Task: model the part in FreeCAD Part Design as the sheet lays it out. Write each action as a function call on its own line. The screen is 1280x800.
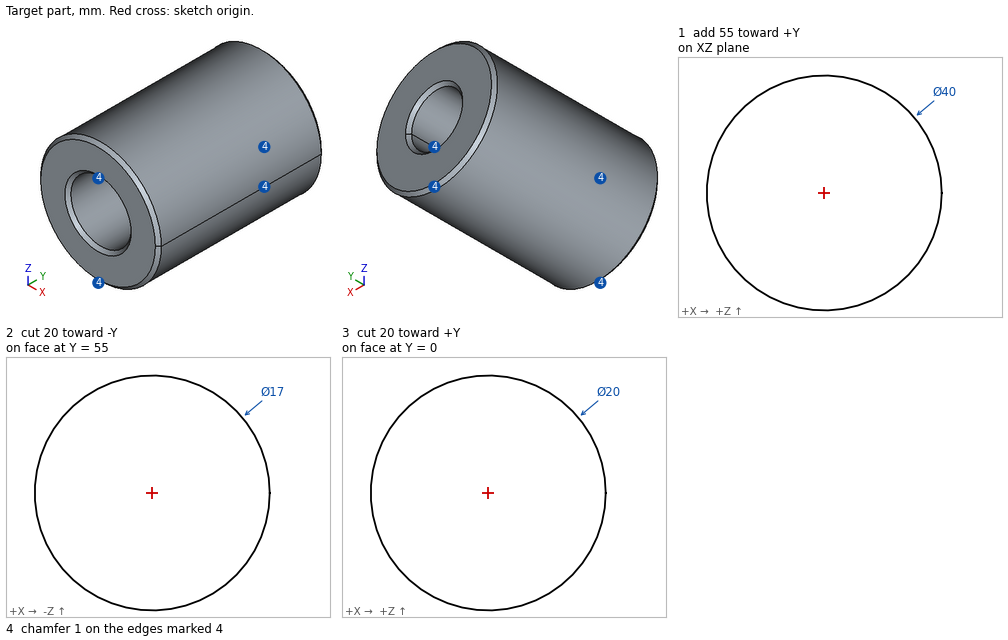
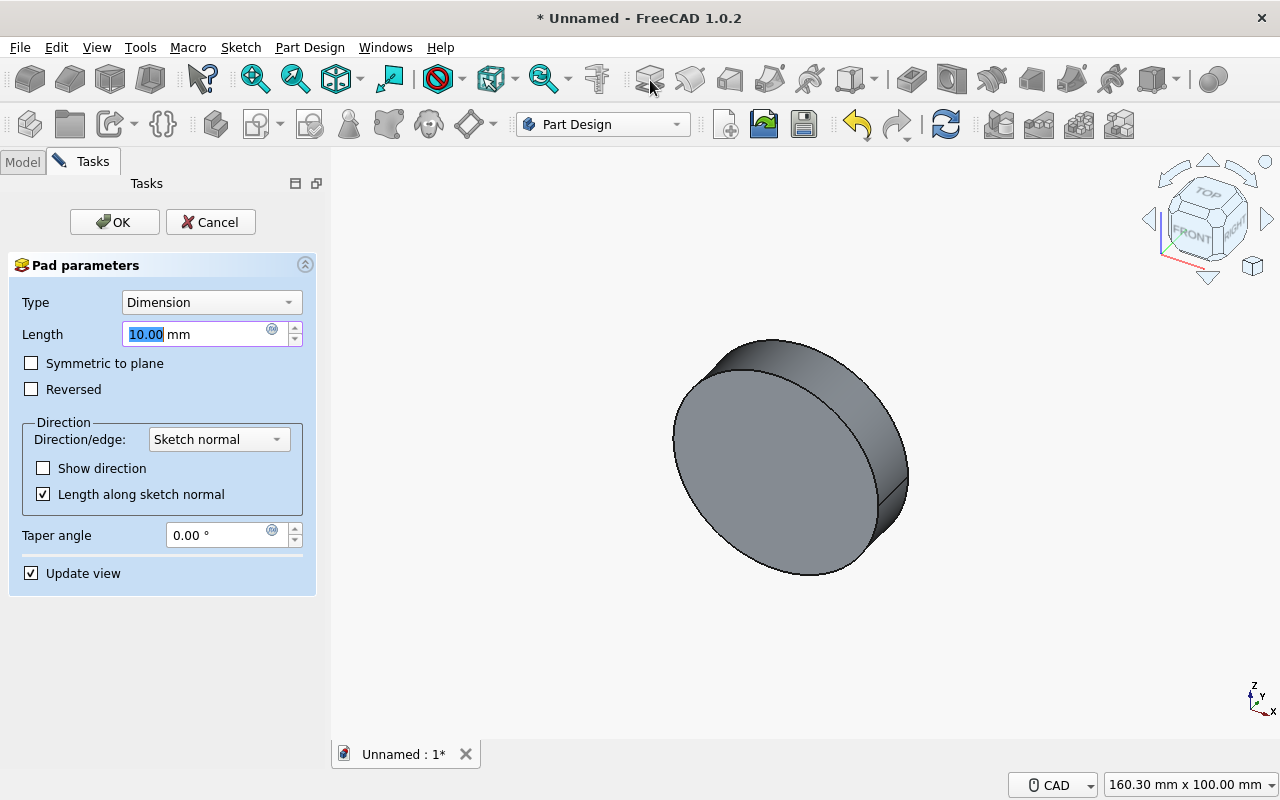
text(55)
key(Tab)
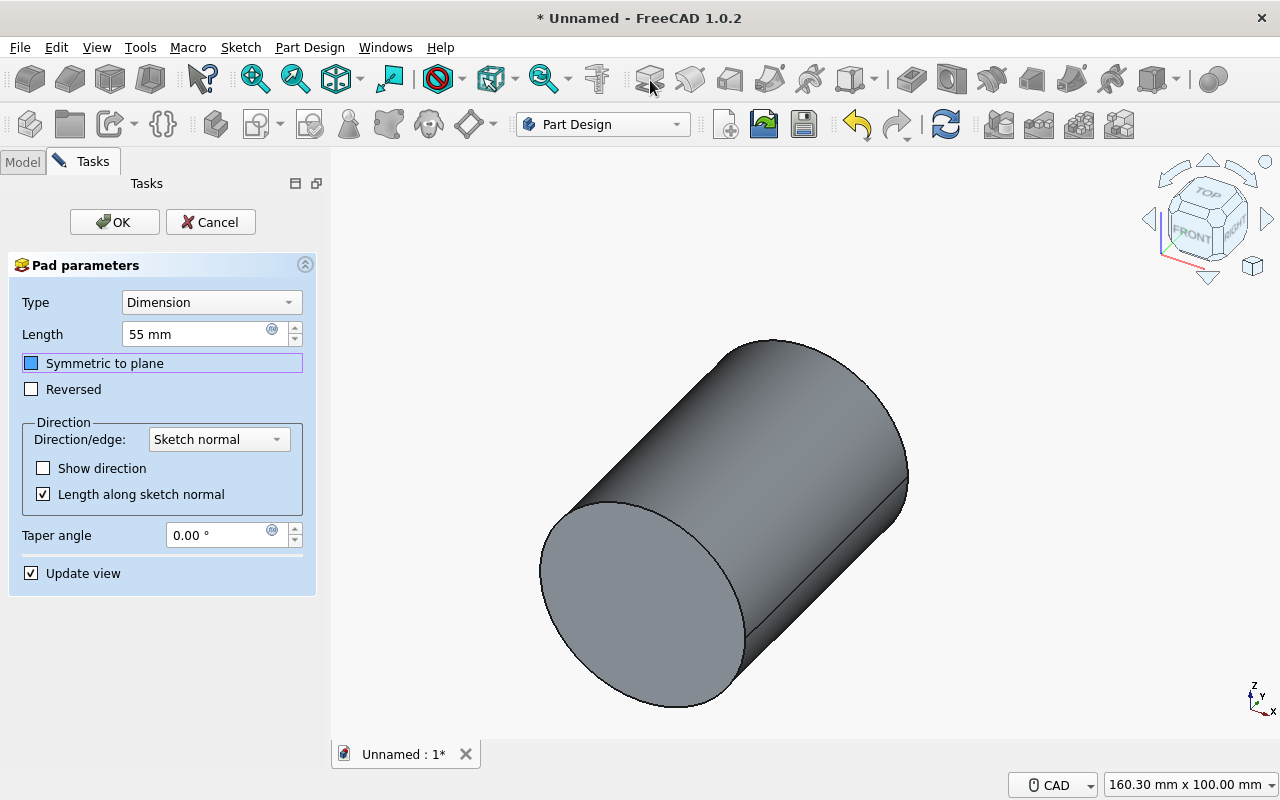
click(30, 389)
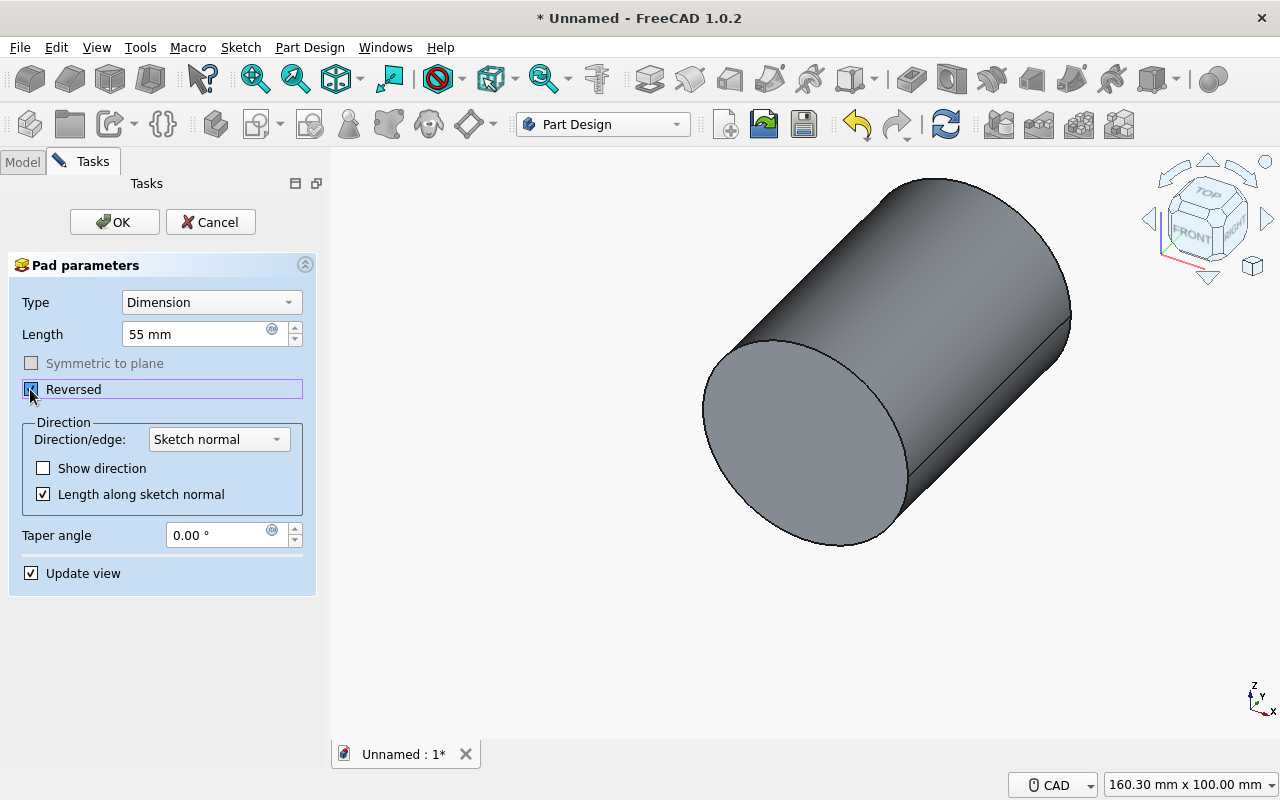
click(115, 222)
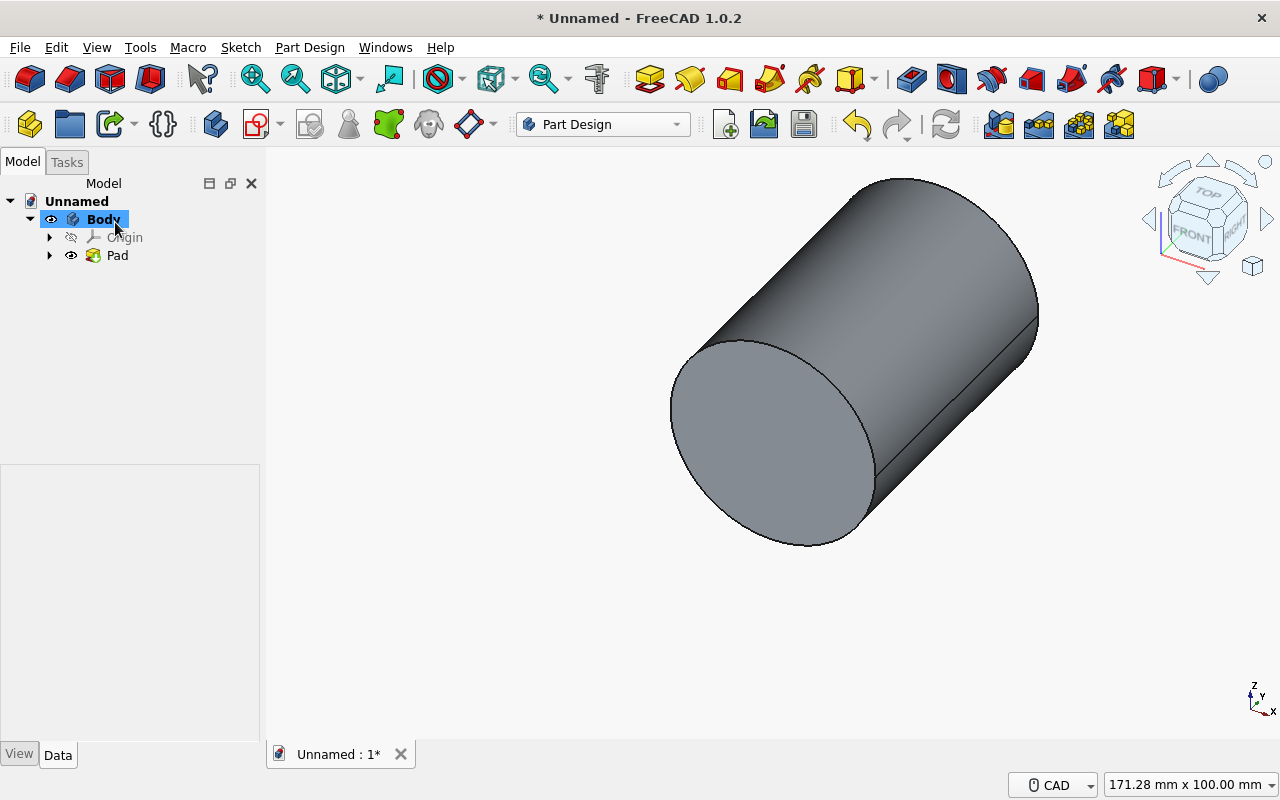
key(4)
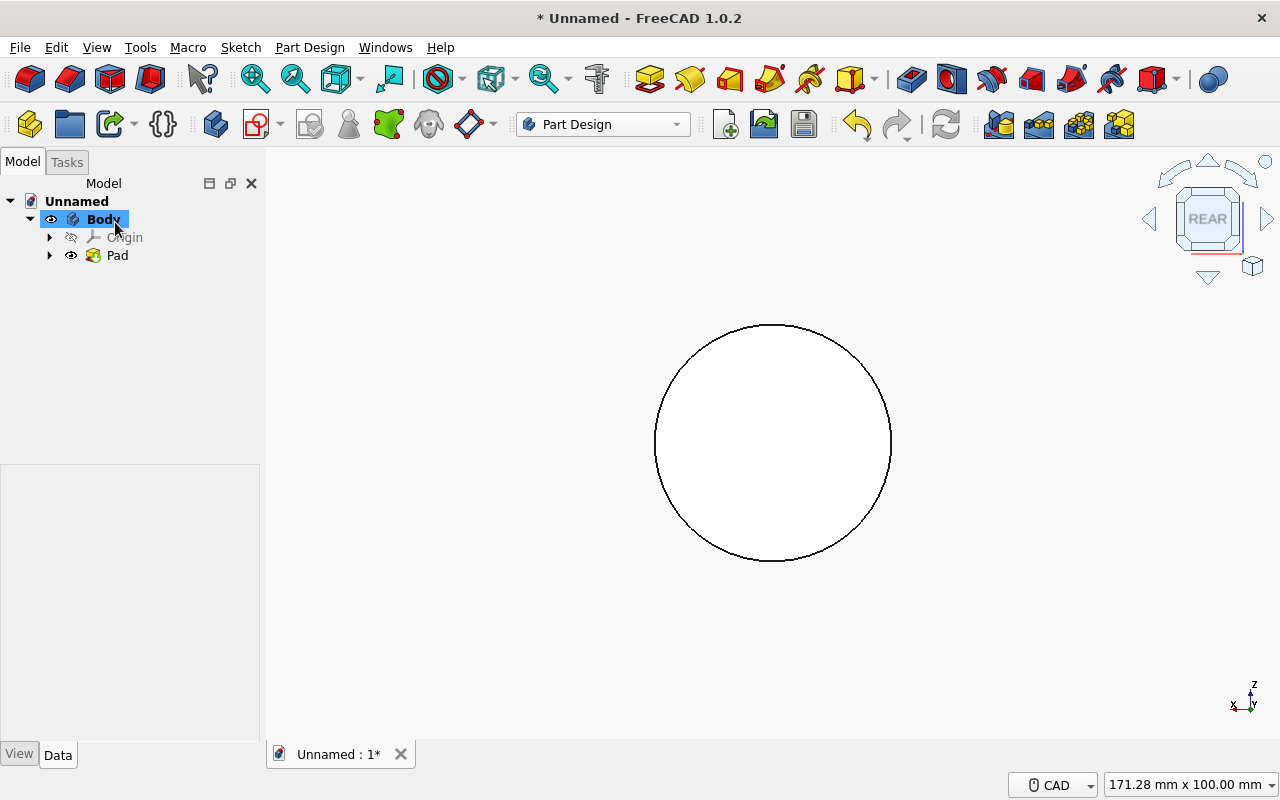
click(256, 80)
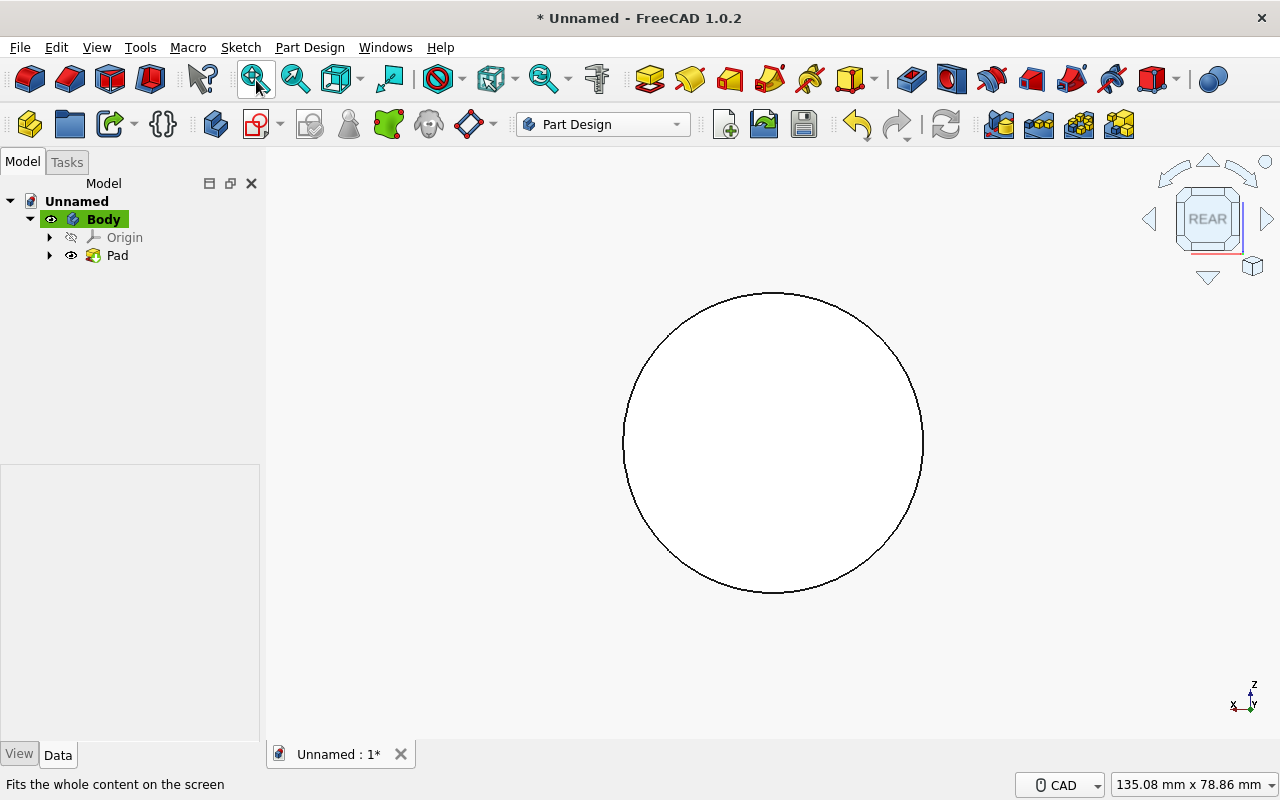
click(773, 442)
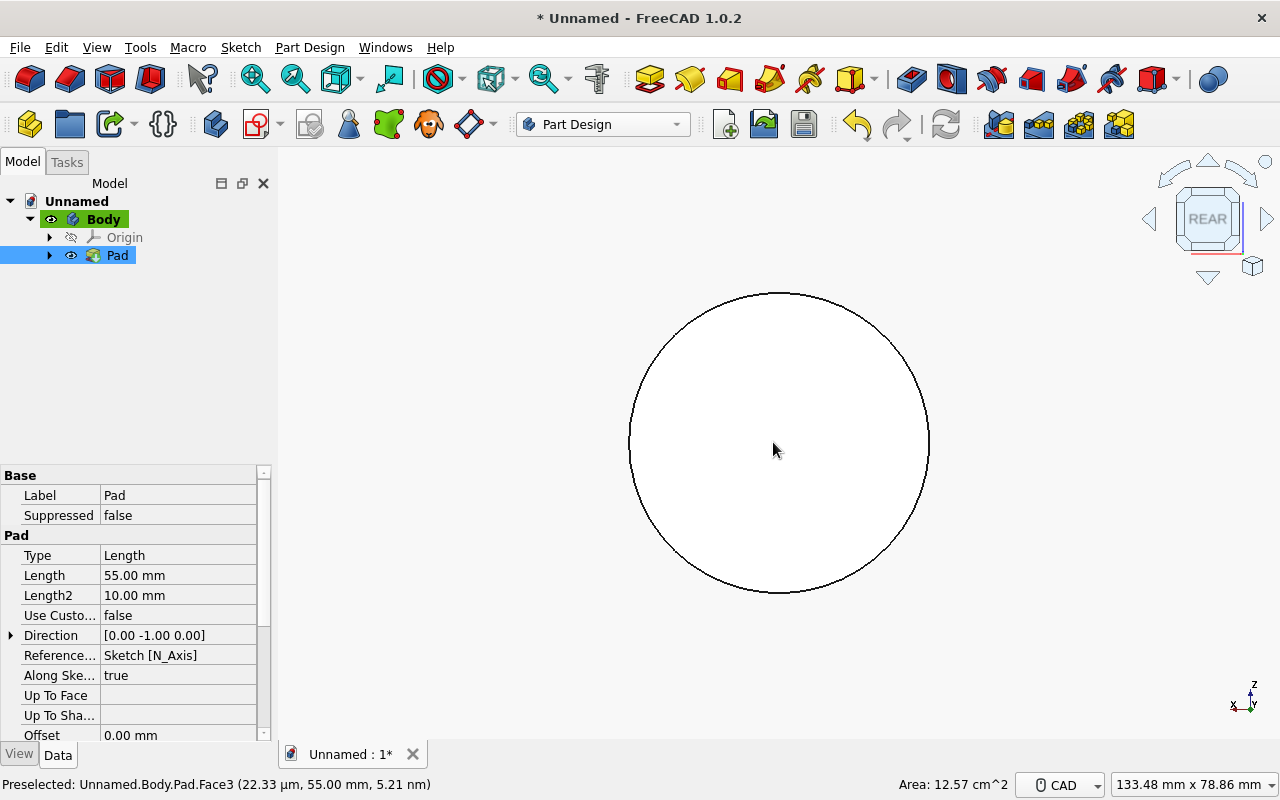
click(256, 124)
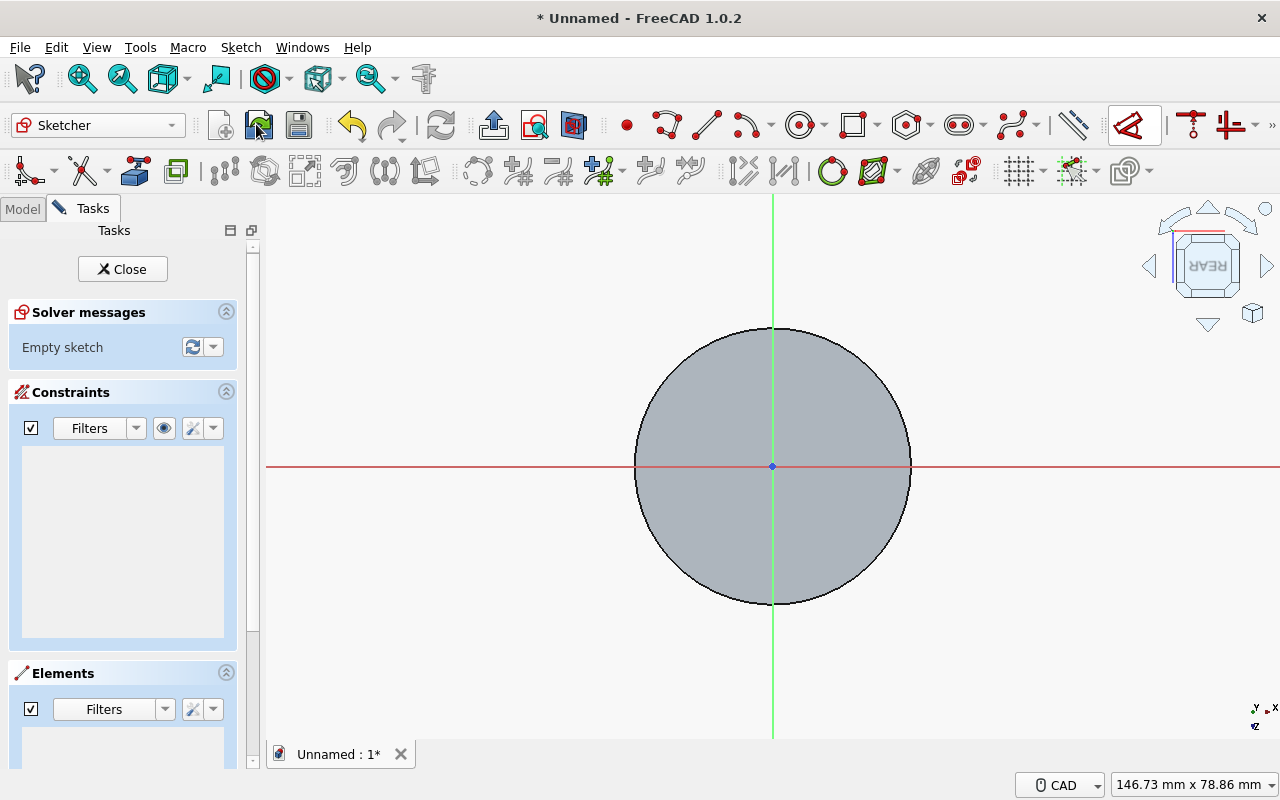
scroll(813, 466, up, 5)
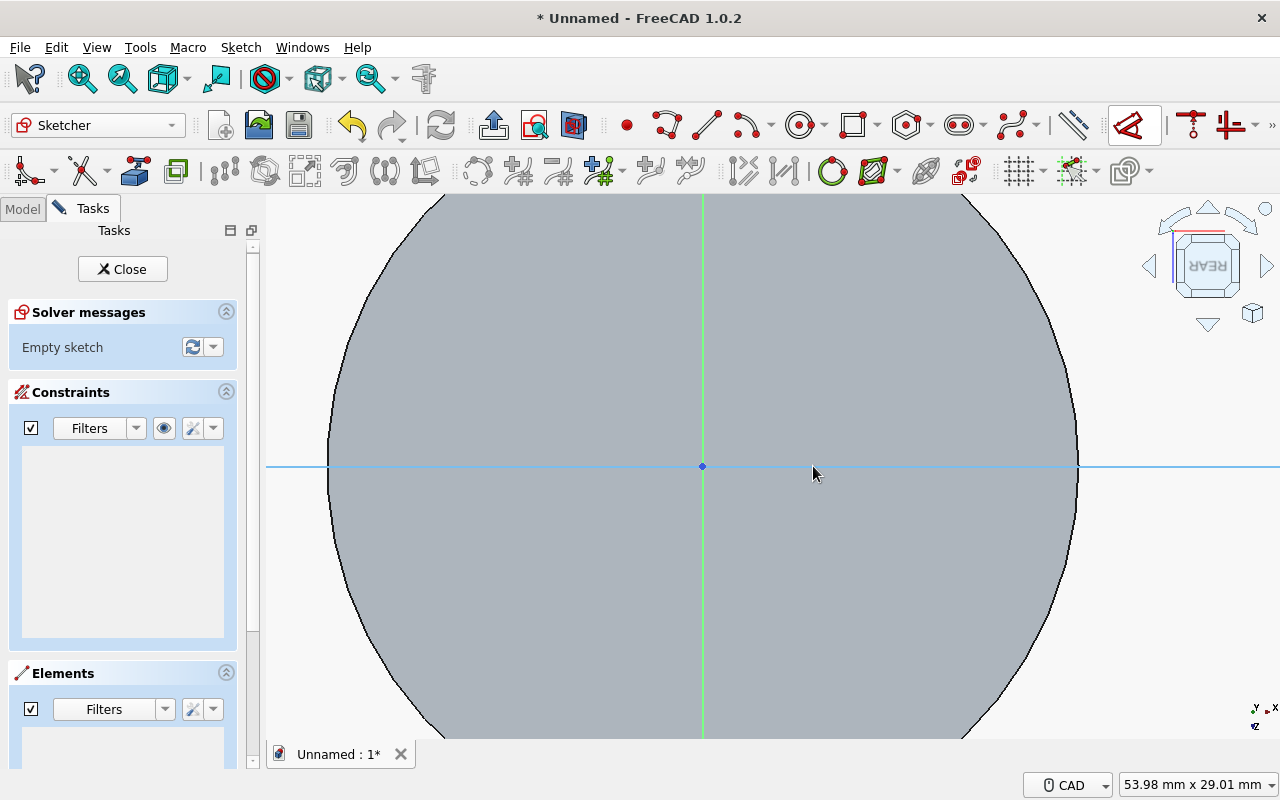
click(800, 126)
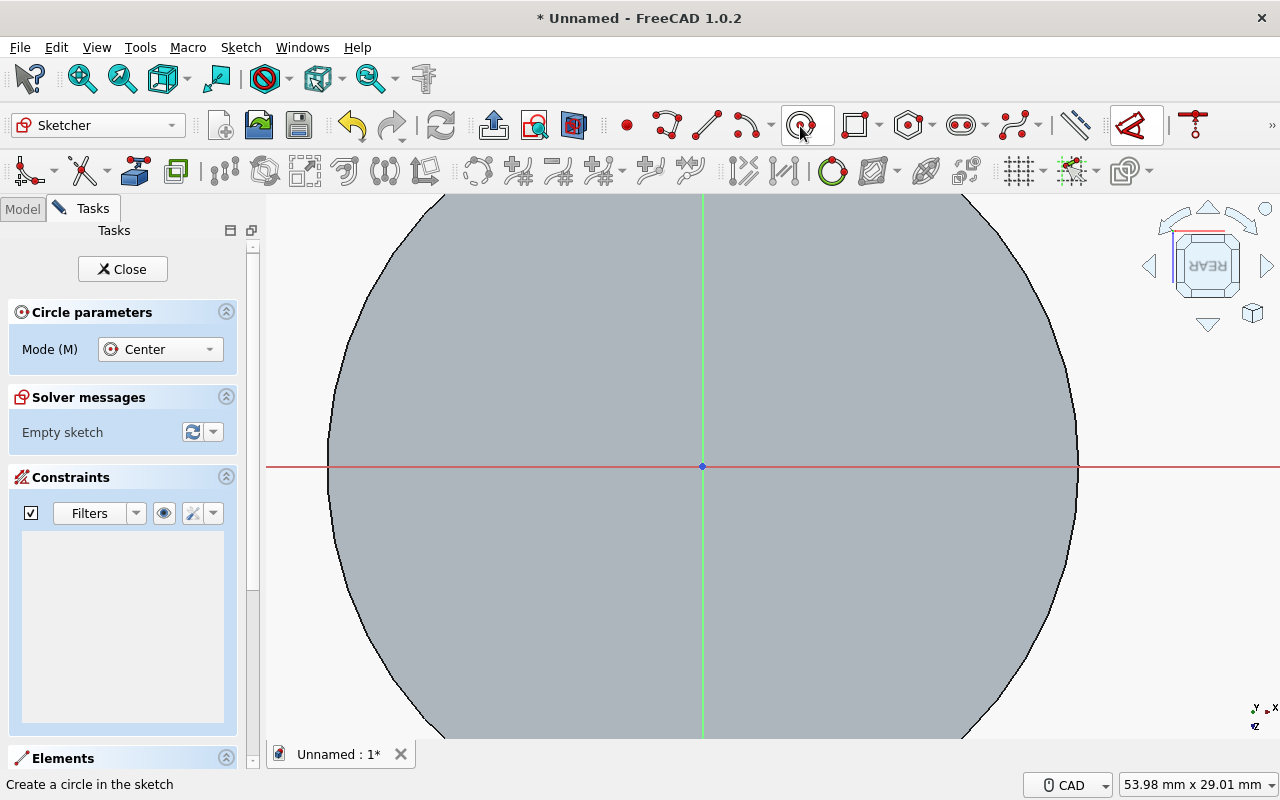
click(703, 466)
move(816, 354)